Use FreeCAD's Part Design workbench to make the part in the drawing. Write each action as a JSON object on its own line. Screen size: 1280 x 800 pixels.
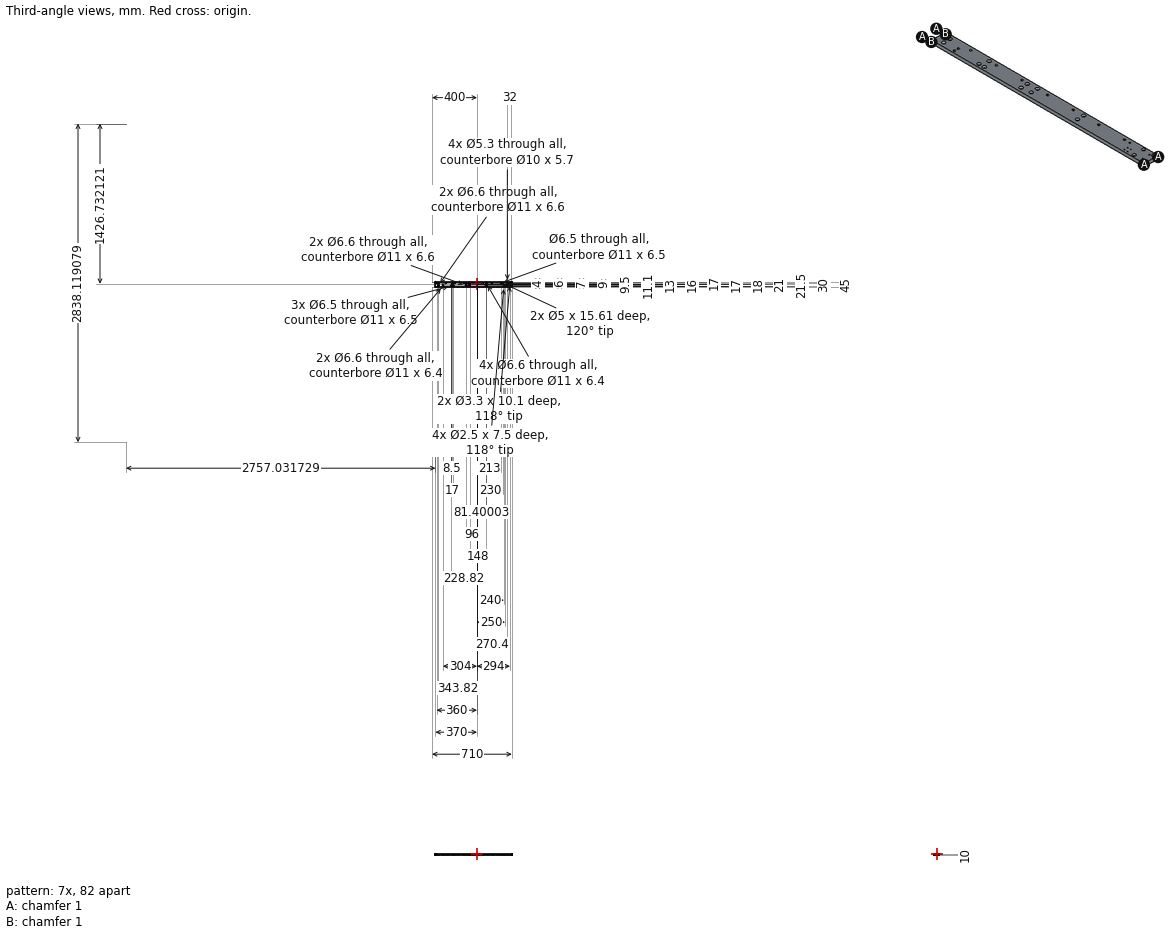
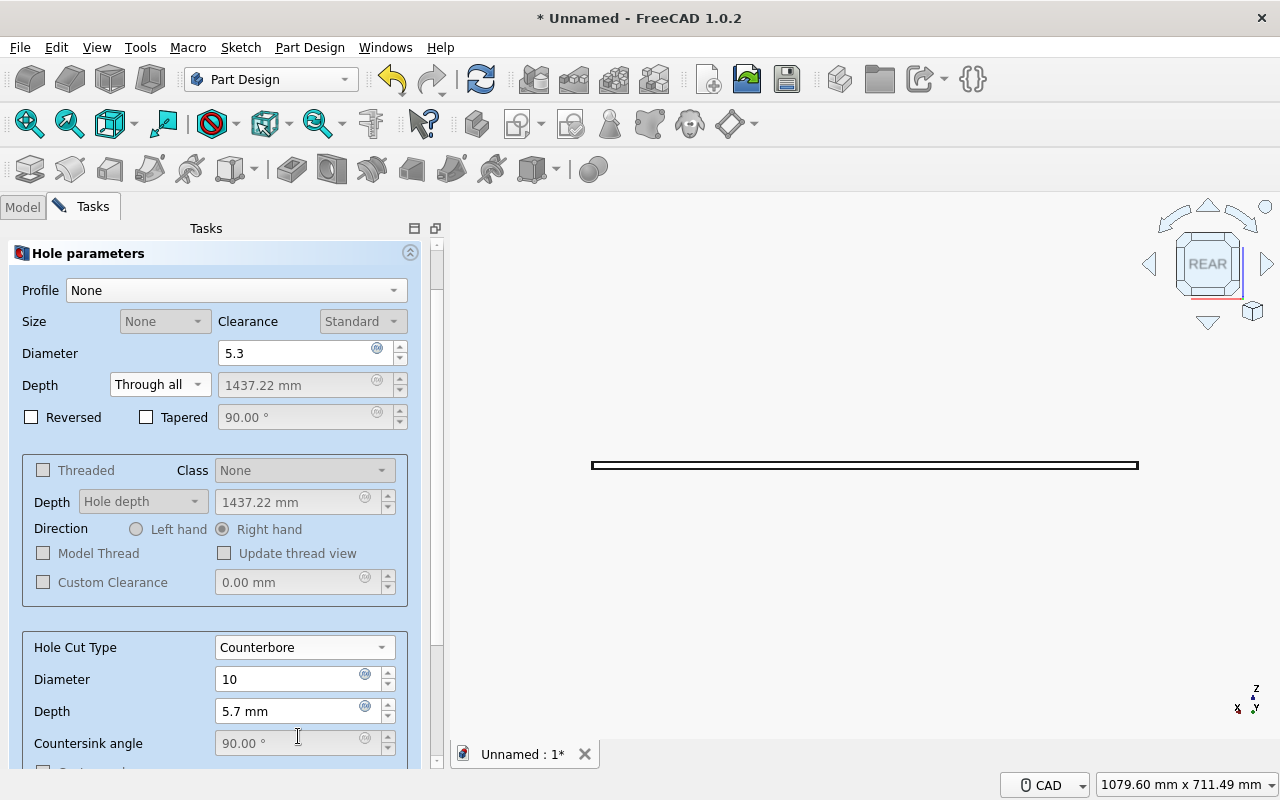
{"action": "scroll", "coordinate": [437, 503], "scroll_direction": "up", "scroll_amount": 2}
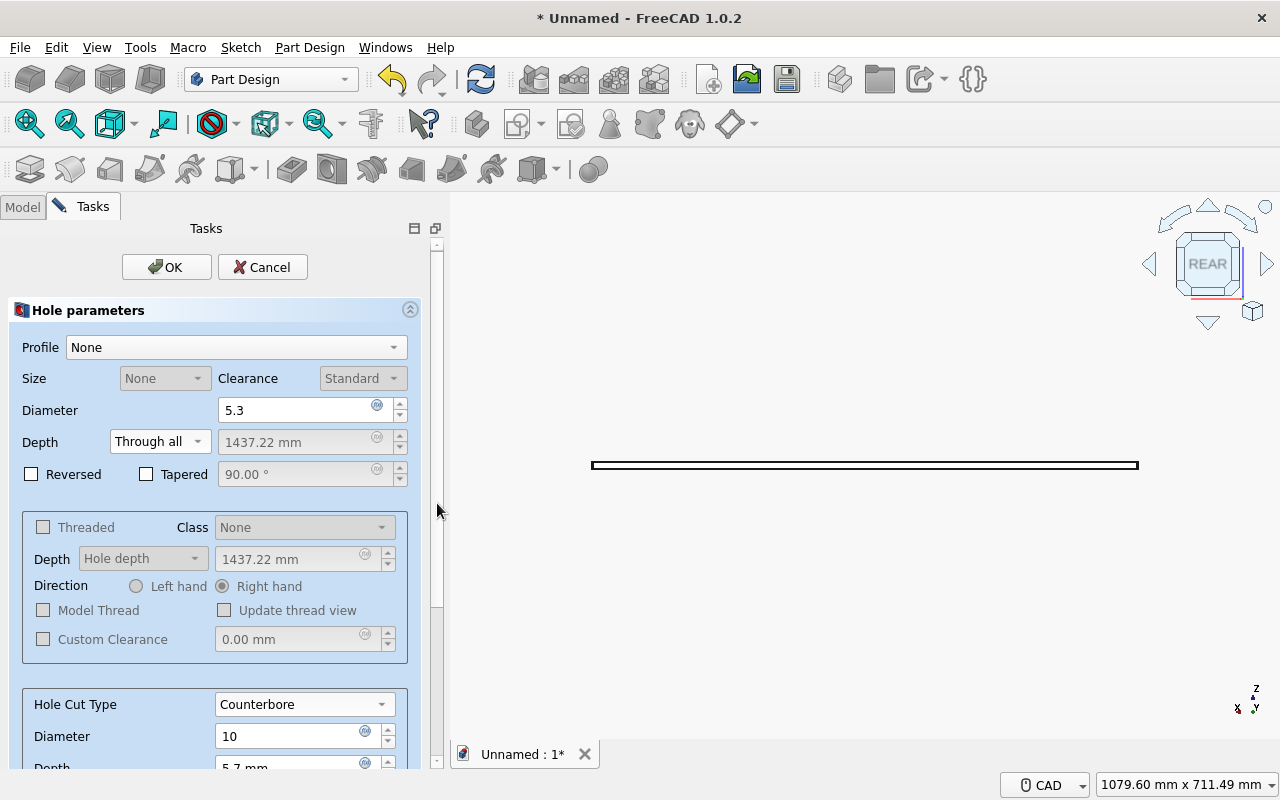
{"action": "left_click", "coordinate": [167, 267]}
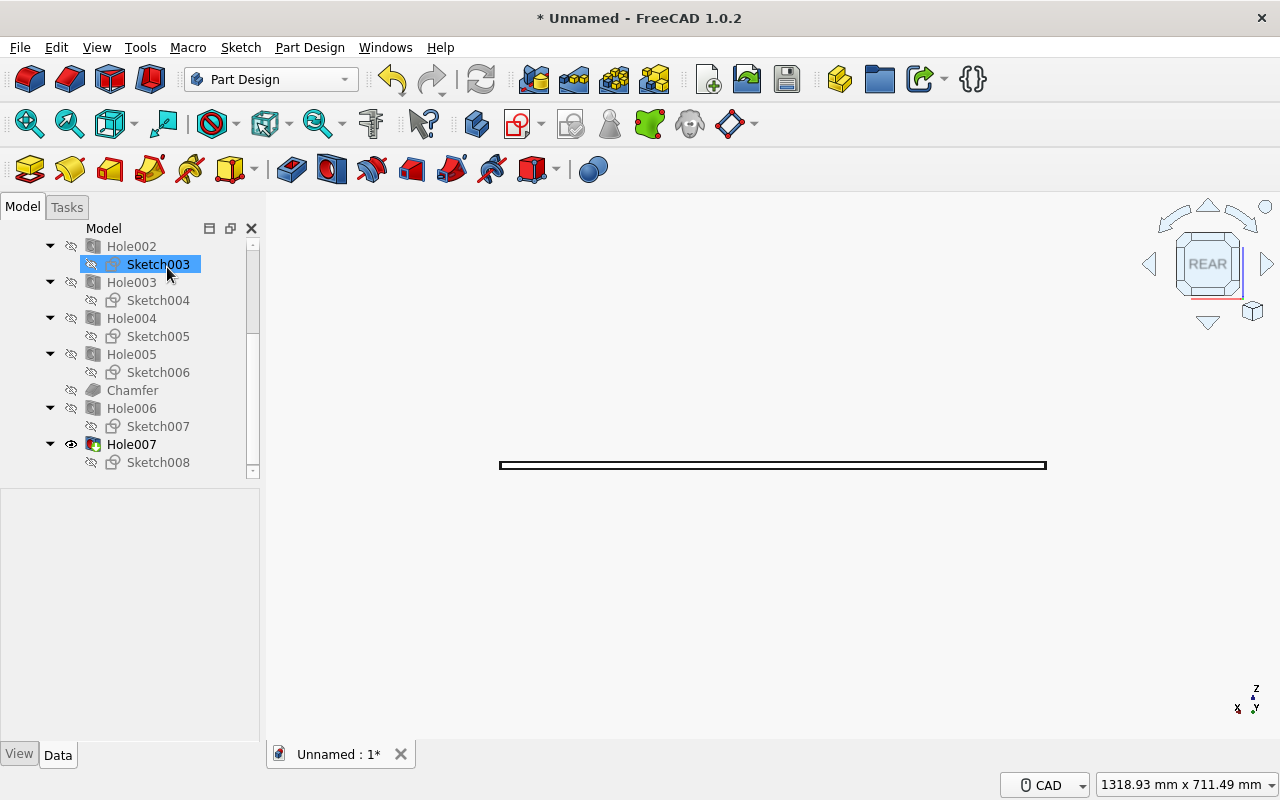
{"action": "left_click", "coordinate": [518, 124]}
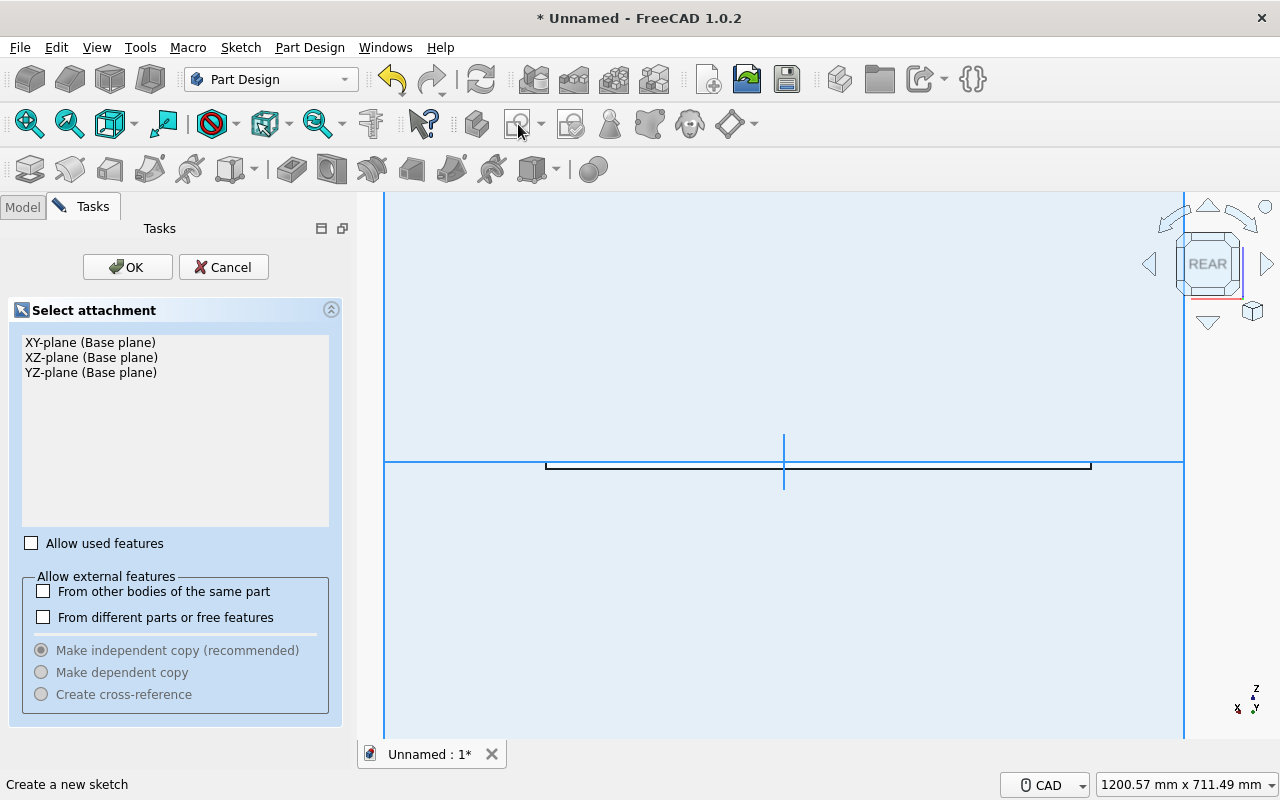
{"action": "left_click", "coordinate": [82, 342]}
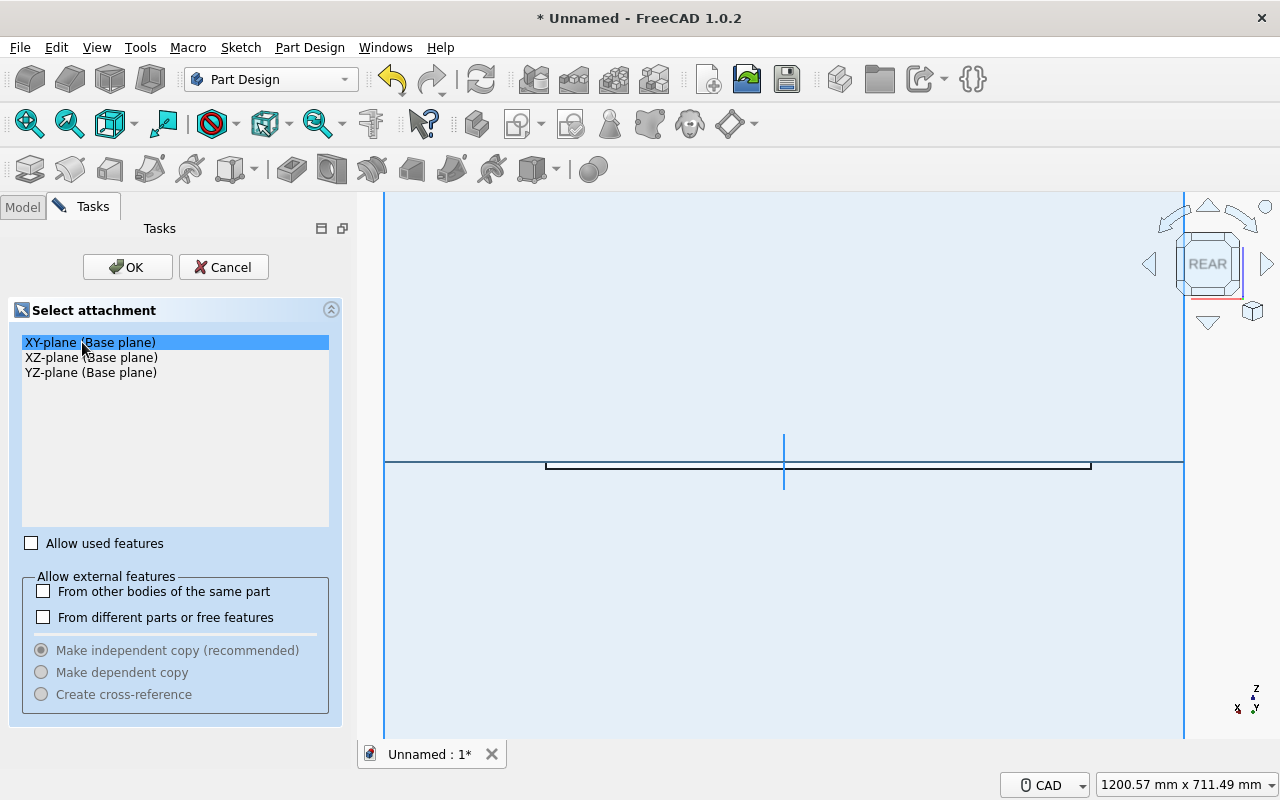
{"action": "left_click", "coordinate": [128, 267]}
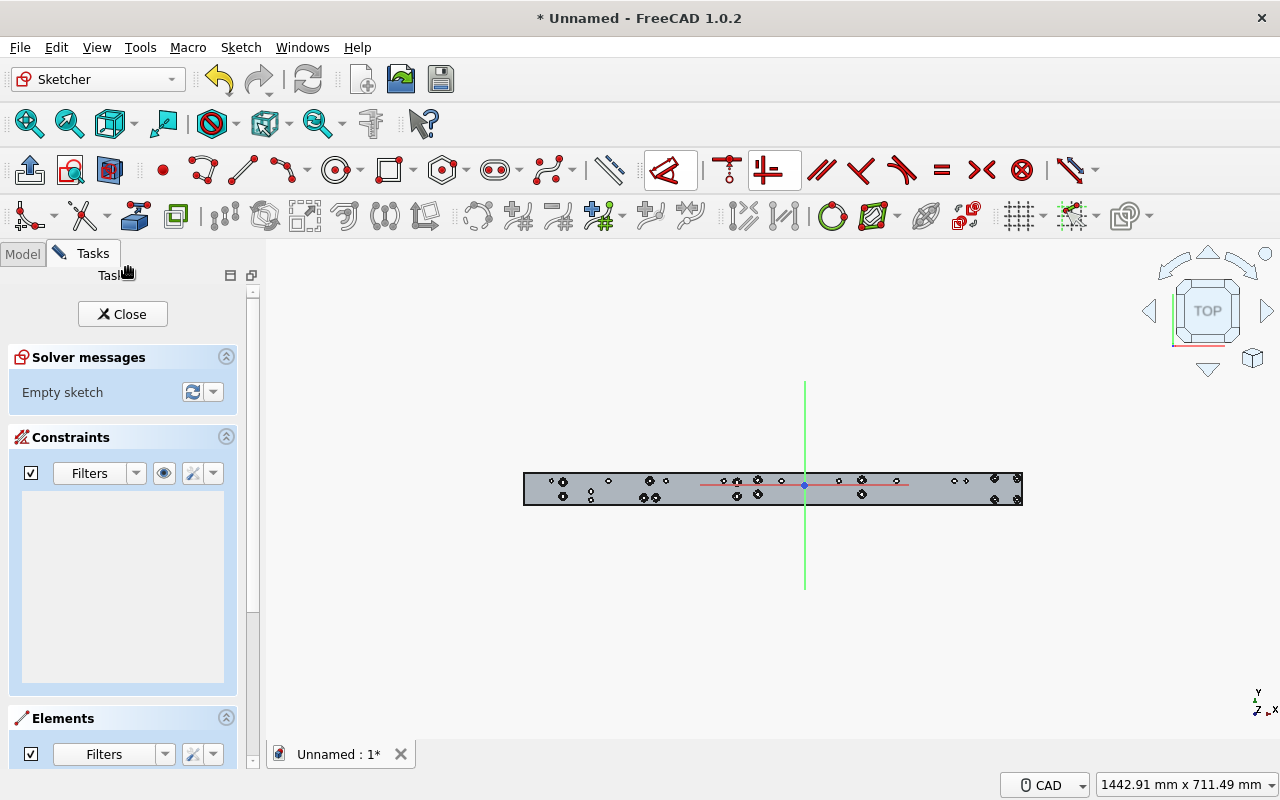
{"action": "scroll", "coordinate": [1027, 490], "scroll_direction": "up", "scroll_amount": 15}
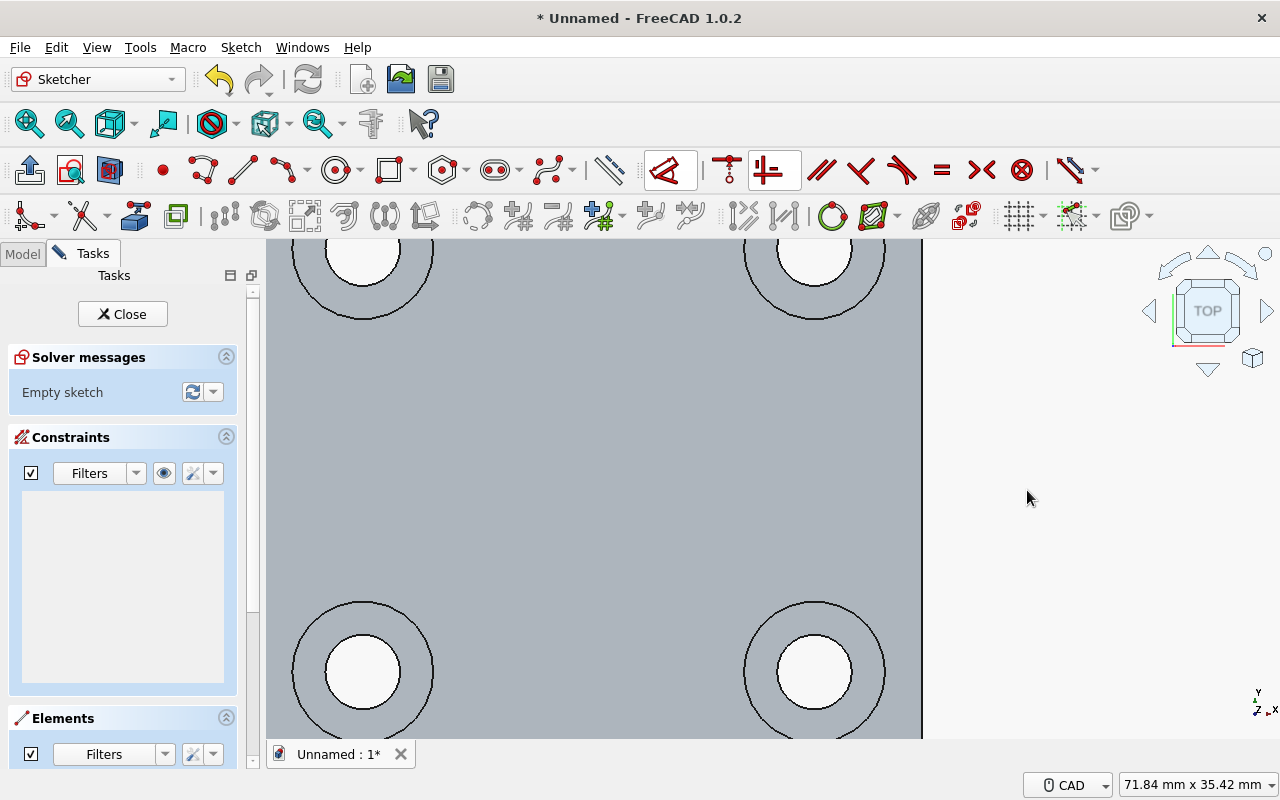
{"action": "left_click", "coordinate": [336, 170]}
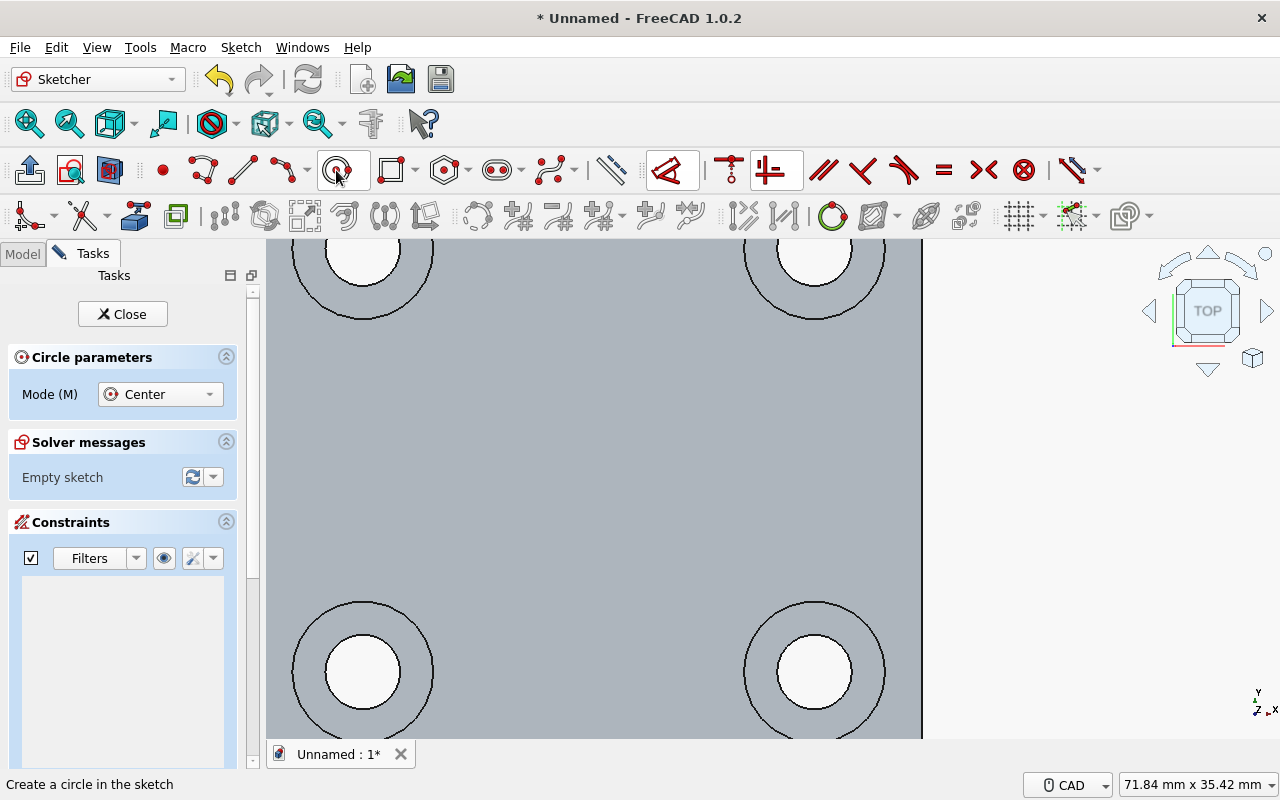
{"action": "left_click", "coordinate": [696, 326]}
{"action": "left_click", "coordinate": [712, 310]}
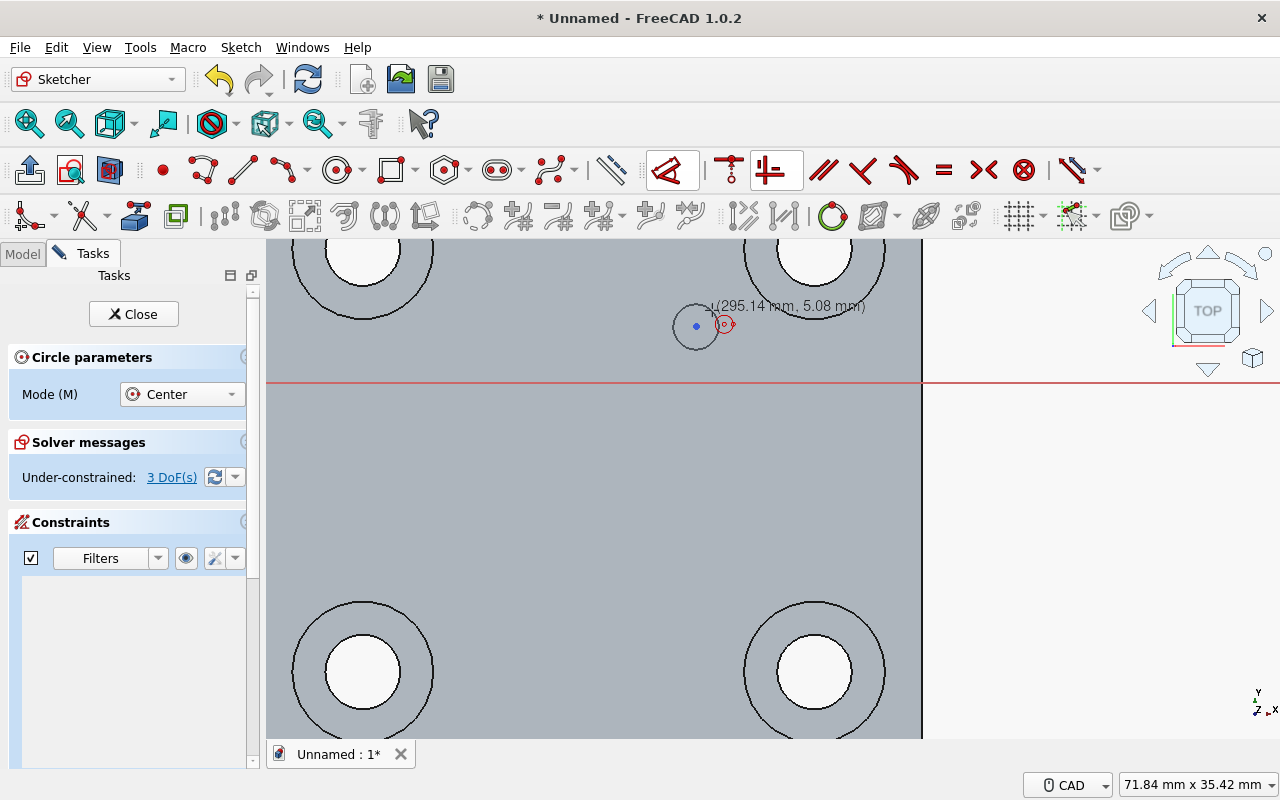
{"action": "left_click", "coordinate": [696, 623]}
{"action": "left_click", "coordinate": [712, 606]}
{"action": "key", "text": "Escape"}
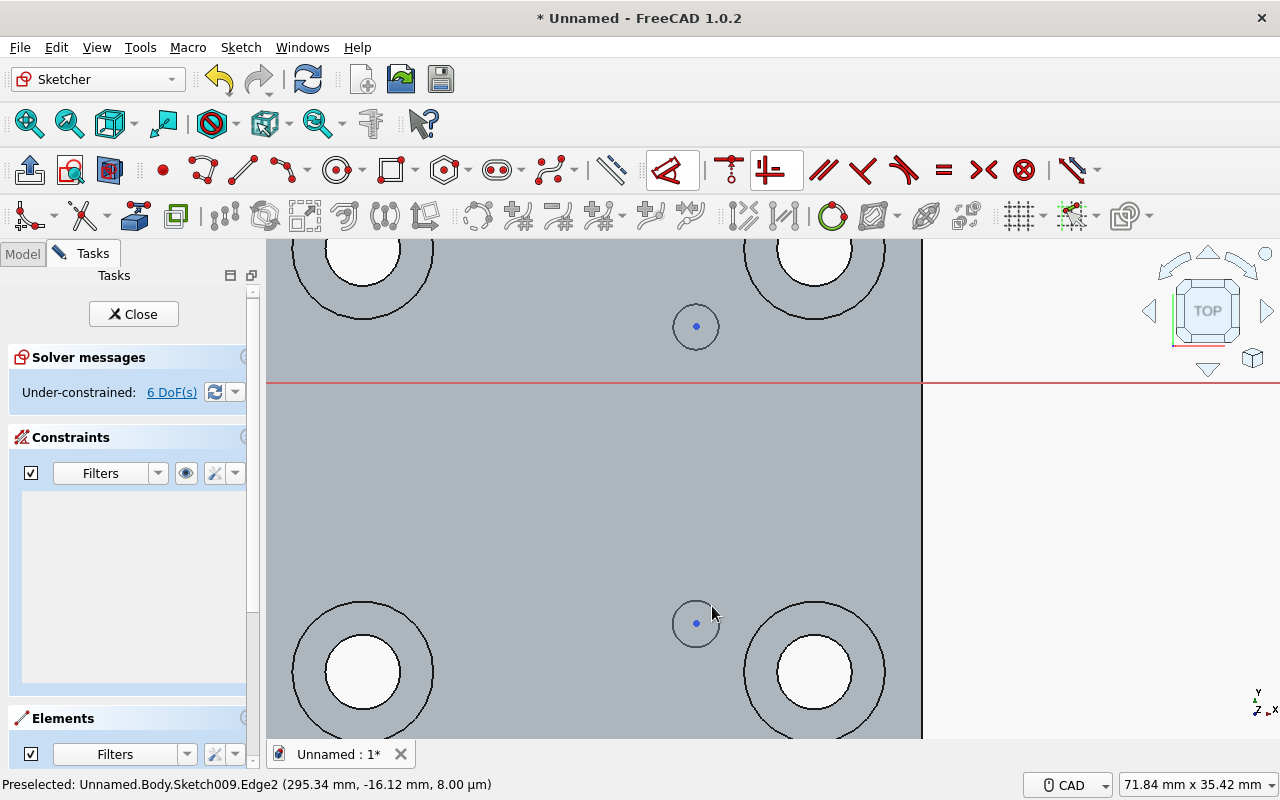
{"action": "left_click", "coordinate": [712, 311]}